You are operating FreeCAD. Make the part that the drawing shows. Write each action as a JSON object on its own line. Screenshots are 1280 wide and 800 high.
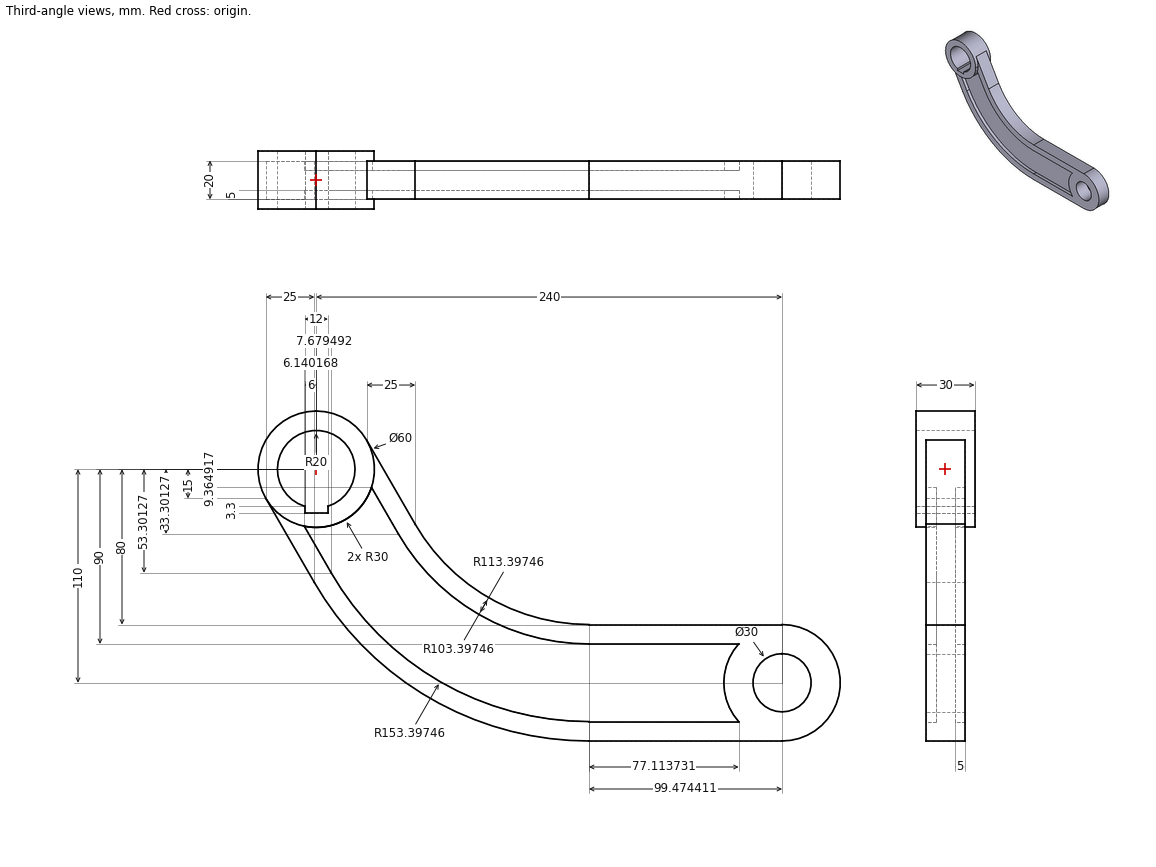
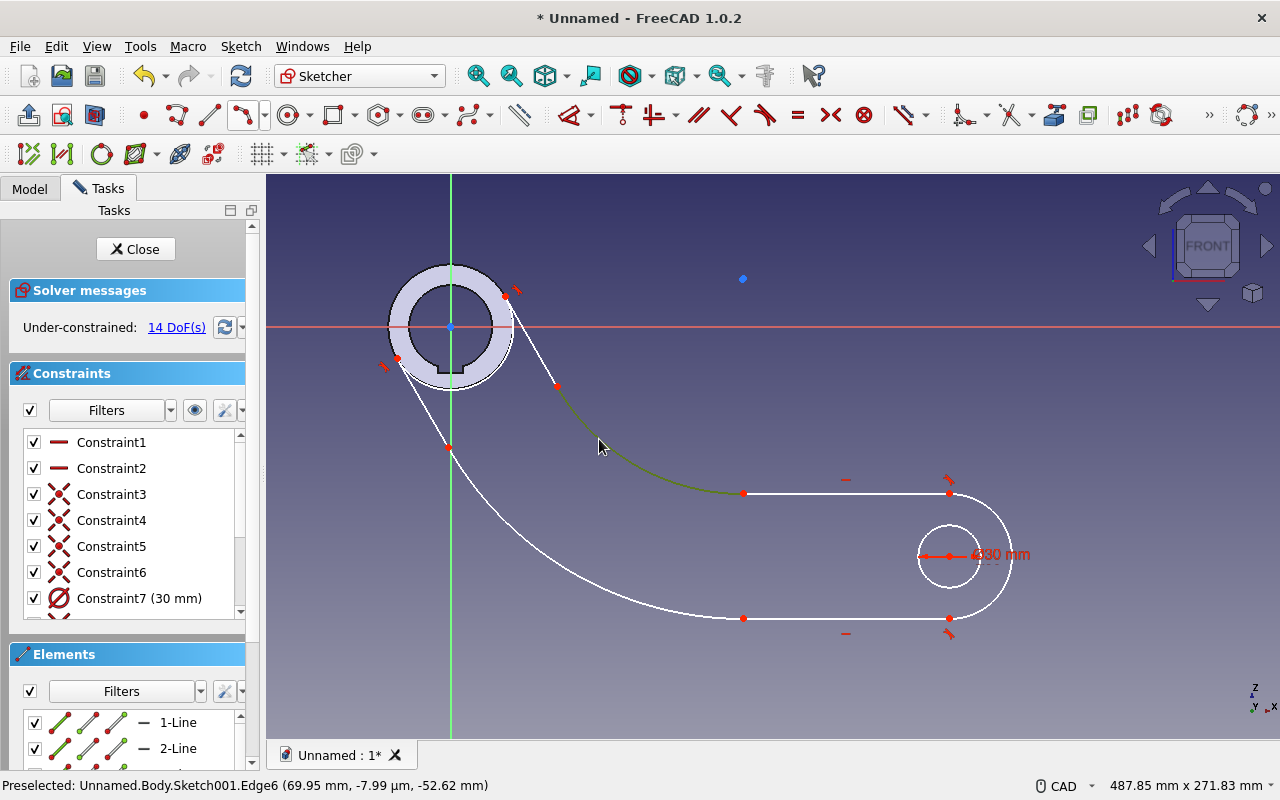
{"action": "left_click", "coordinate": [515, 531]}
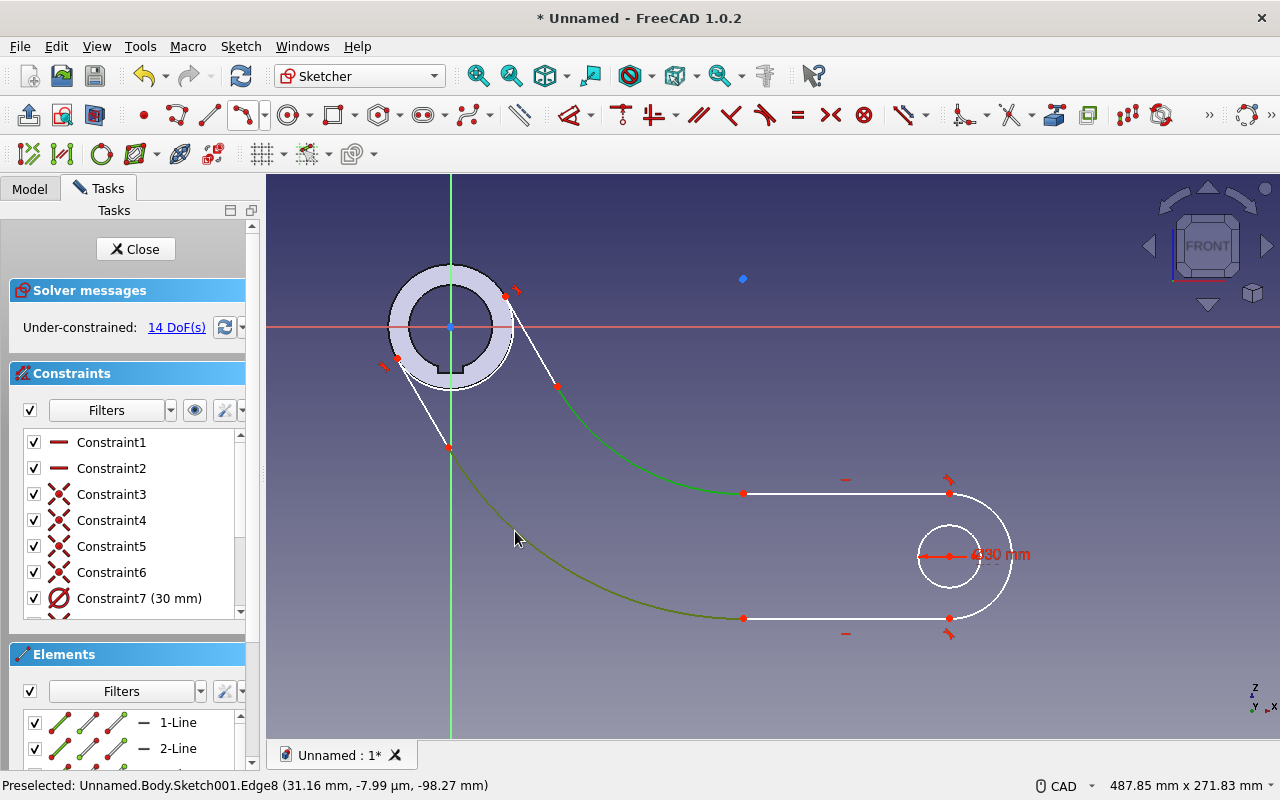
{"action": "left_click", "coordinate": [621, 116]}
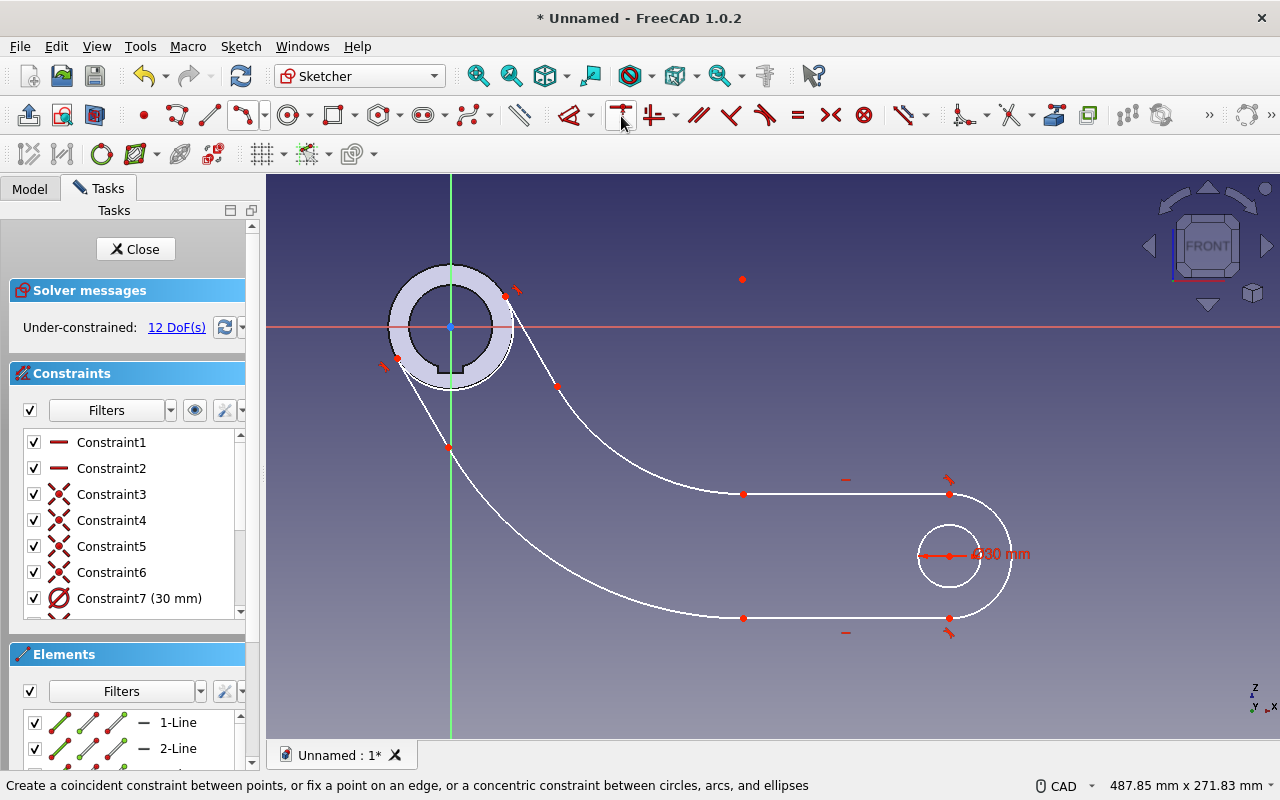
{"action": "scroll", "coordinate": [451, 327], "scroll_direction": "up", "scroll_amount": 2}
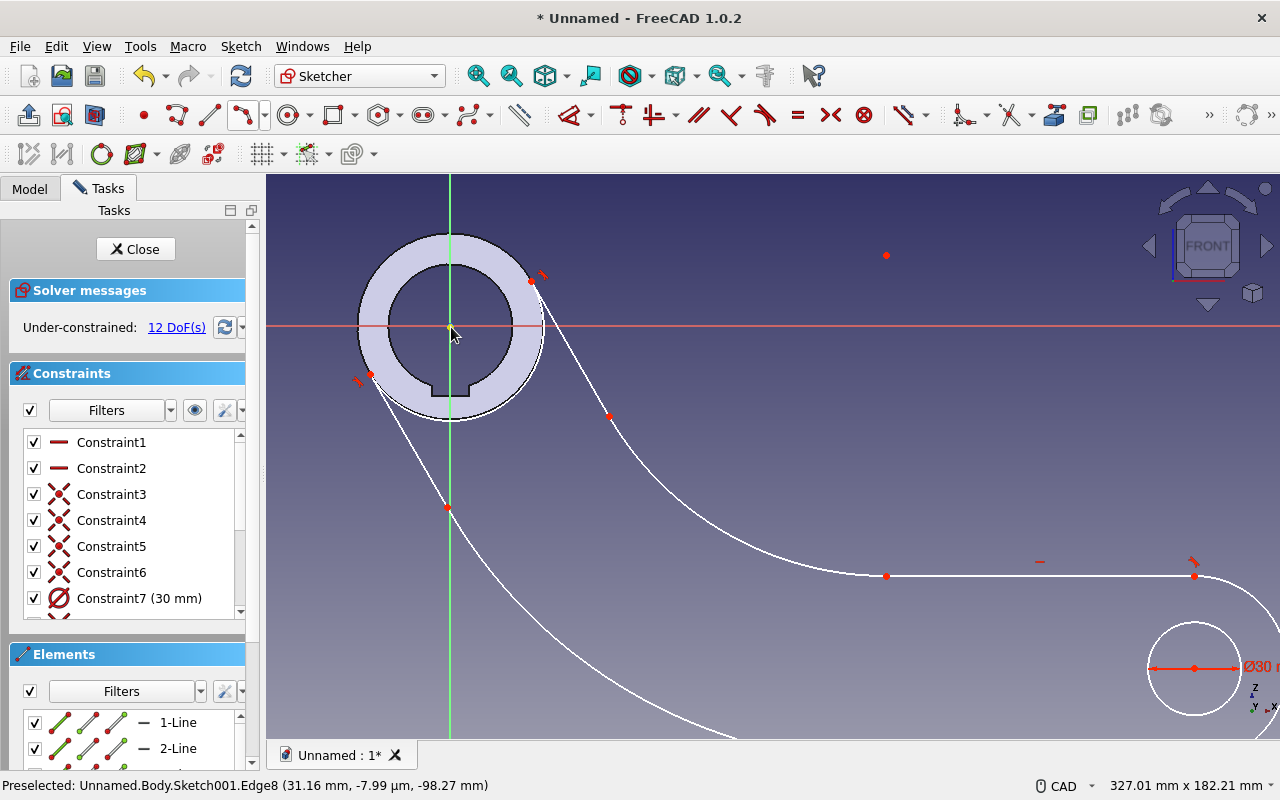
{"action": "left_click_drag", "start_coordinate": [440, 316], "coordinate": [461, 338]}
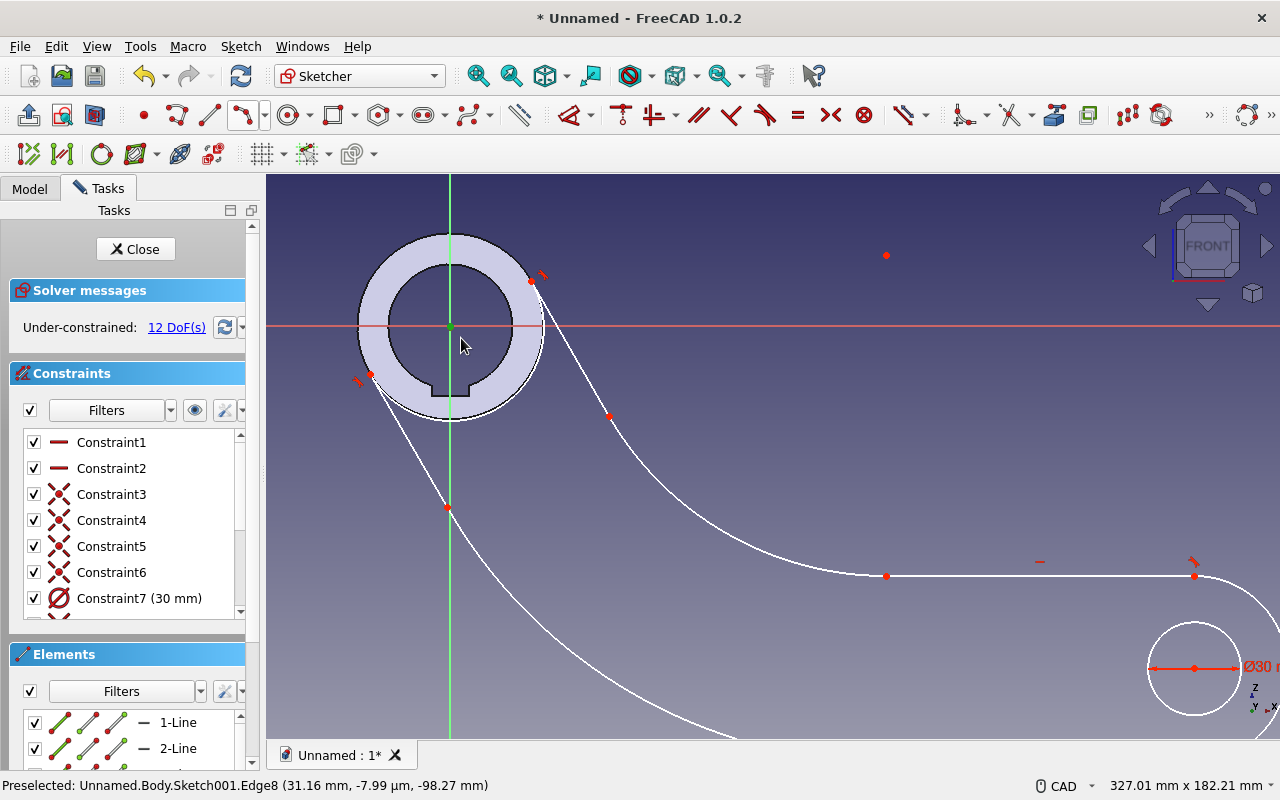
{"action": "left_click", "coordinate": [621, 116]}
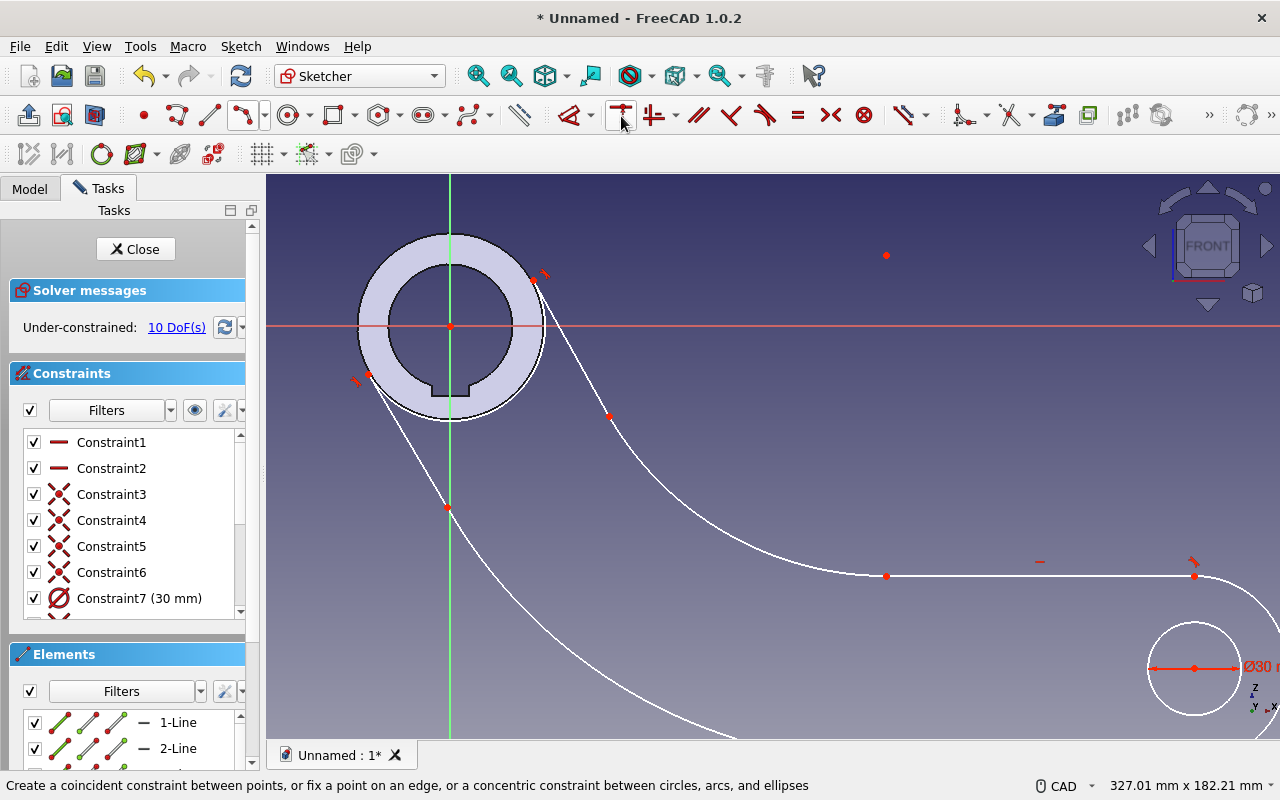
{"action": "scroll", "coordinate": [441, 421], "scroll_direction": "up", "scroll_amount": 2}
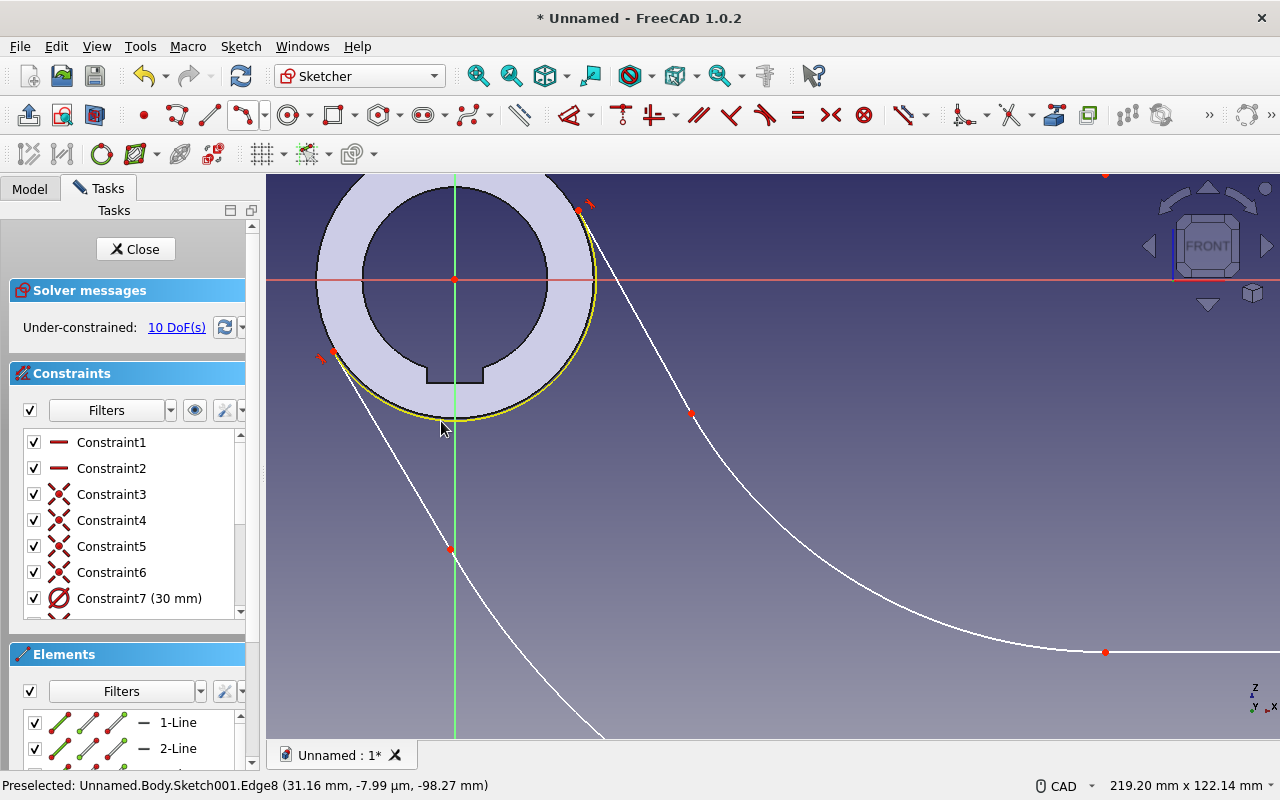
{"action": "left_click", "coordinate": [441, 420]}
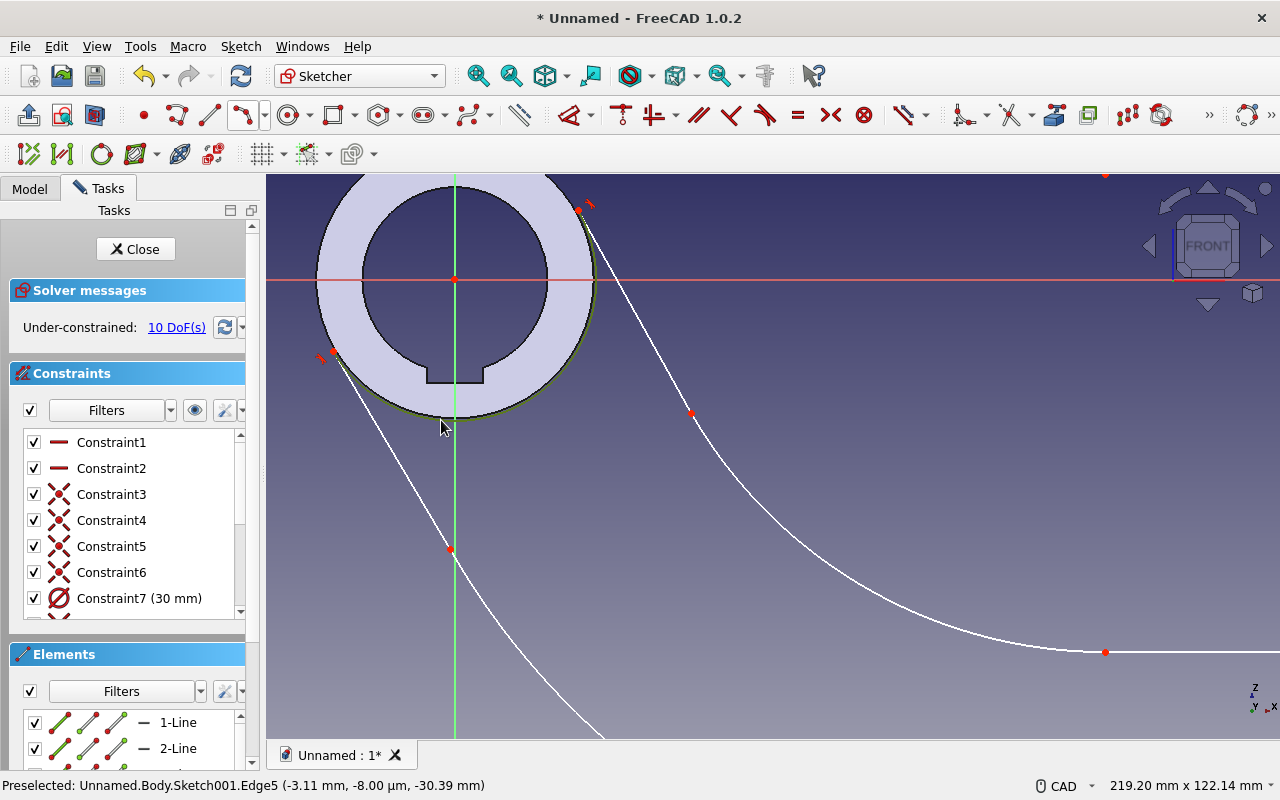
{"action": "scroll", "coordinate": [448, 365], "scroll_direction": "down", "scroll_amount": 4}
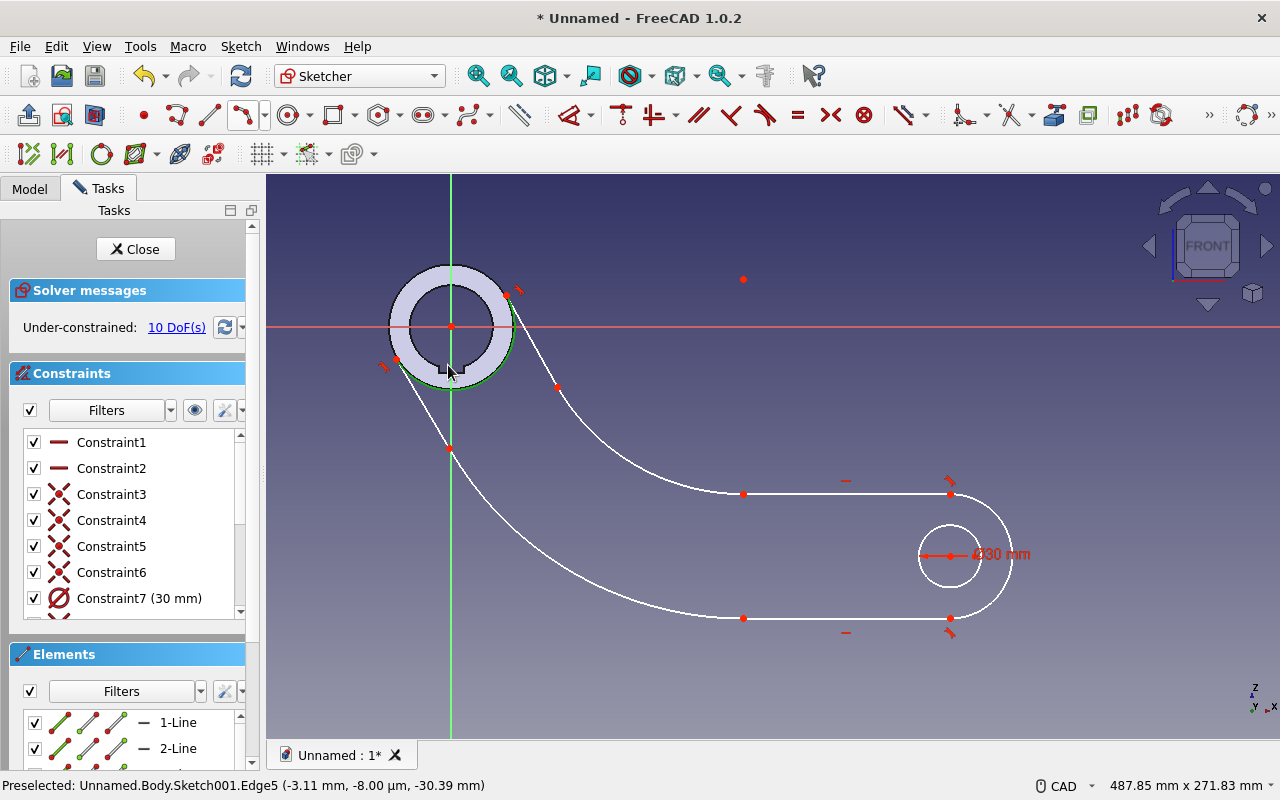
{"action": "left_click", "coordinate": [1000, 593]}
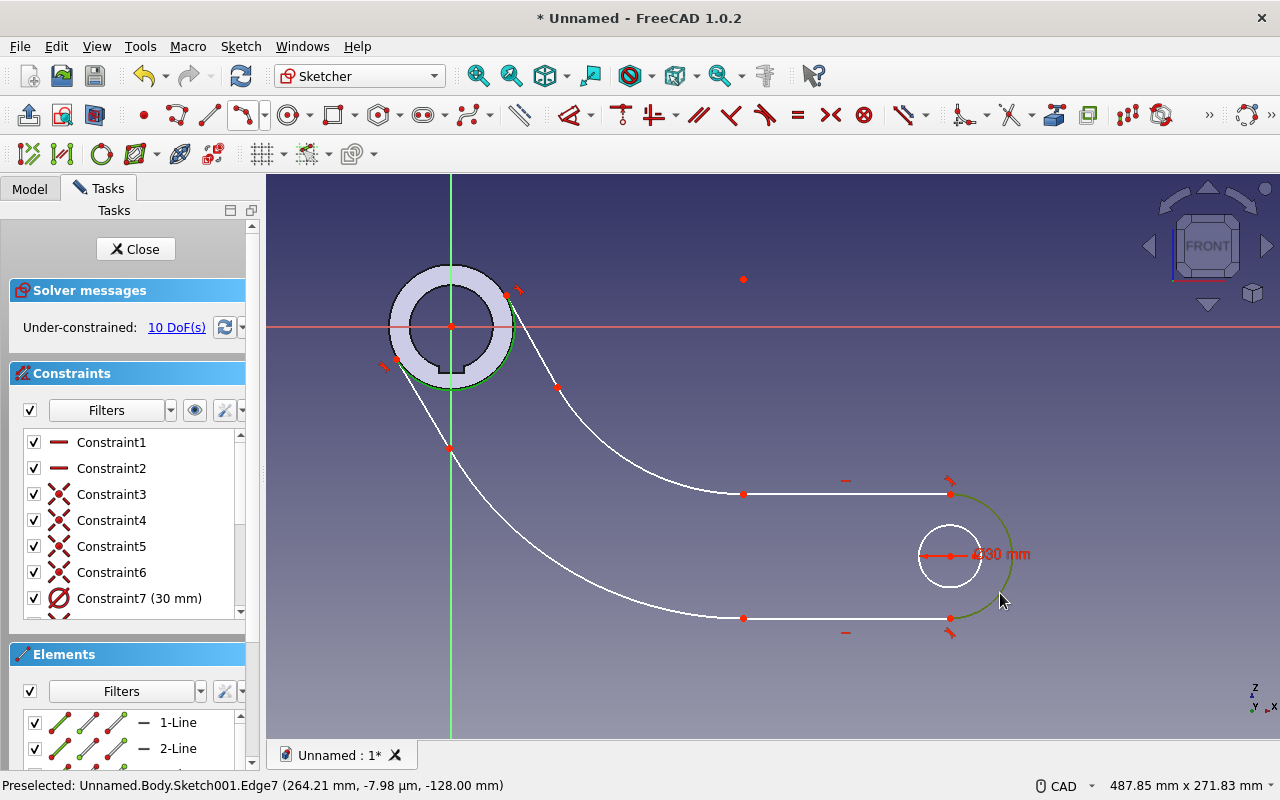
{"action": "key", "text": "e"}